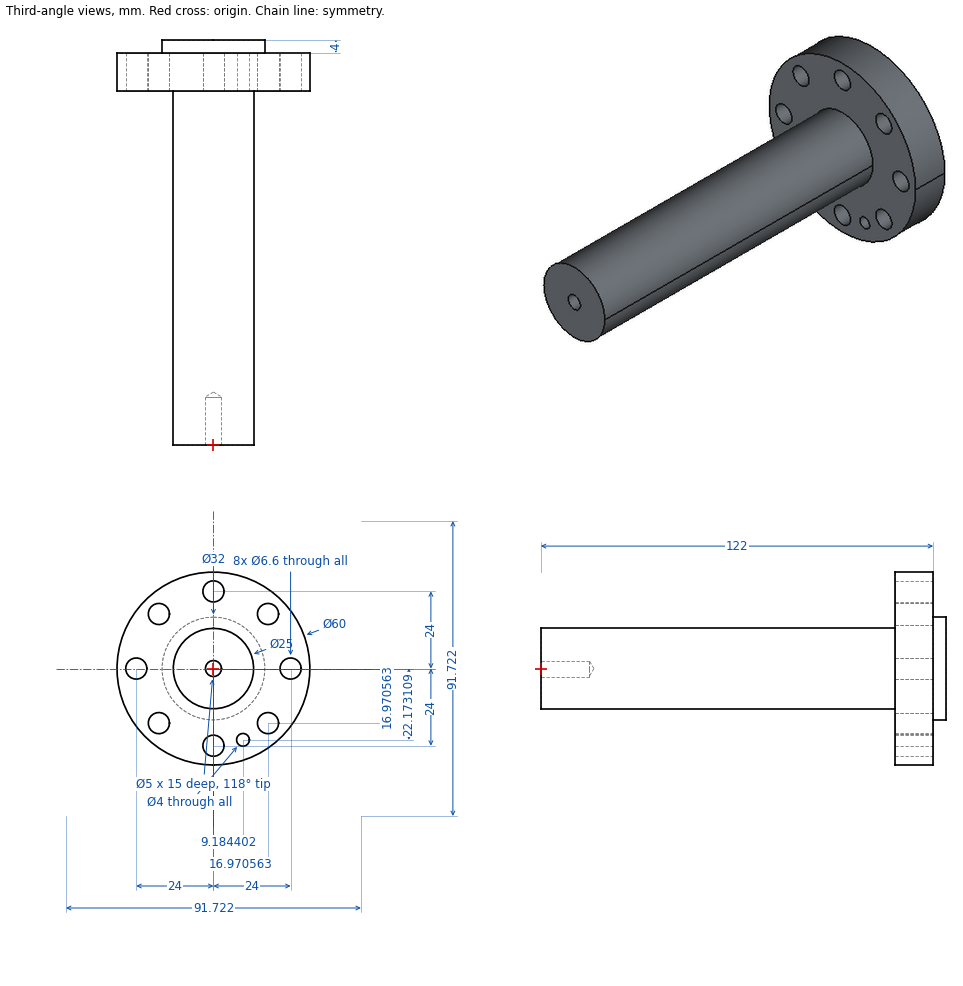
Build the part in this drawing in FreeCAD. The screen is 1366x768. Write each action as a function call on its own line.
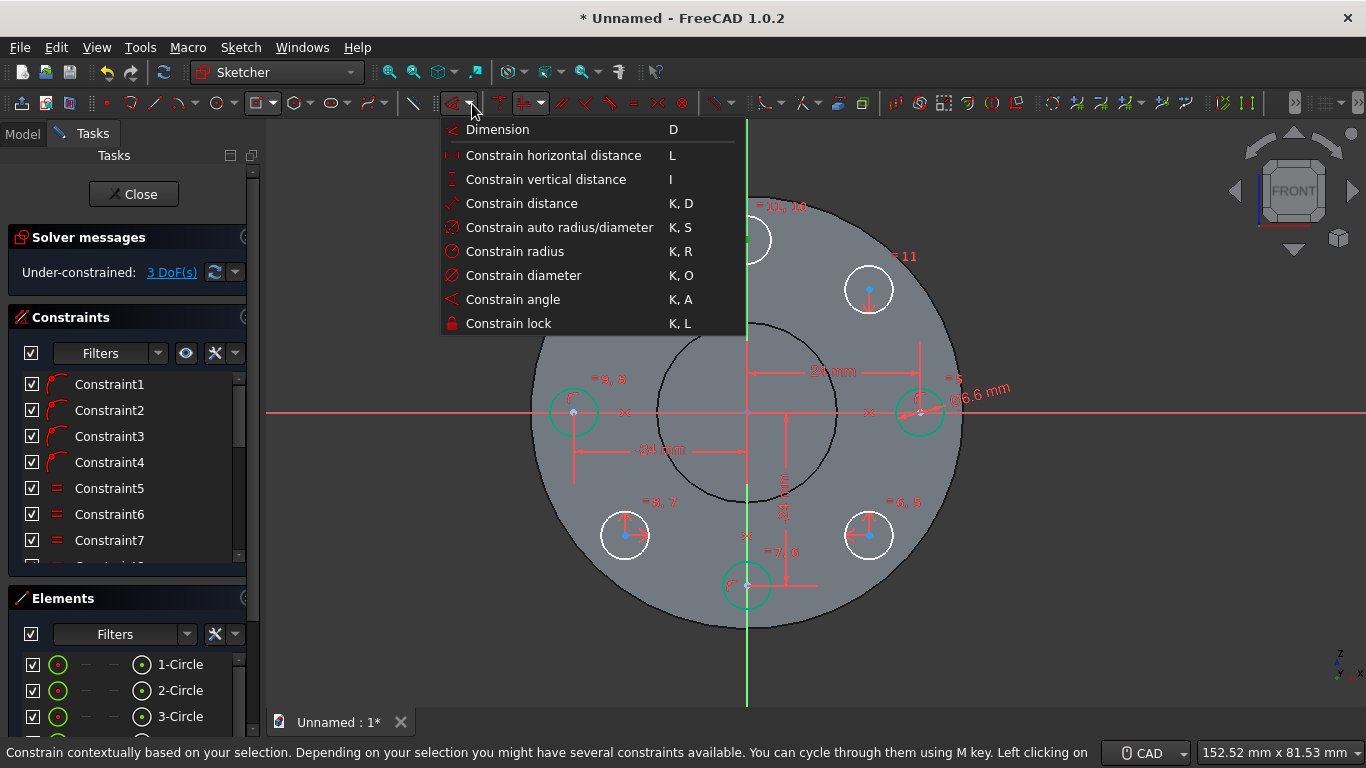
click(593, 179)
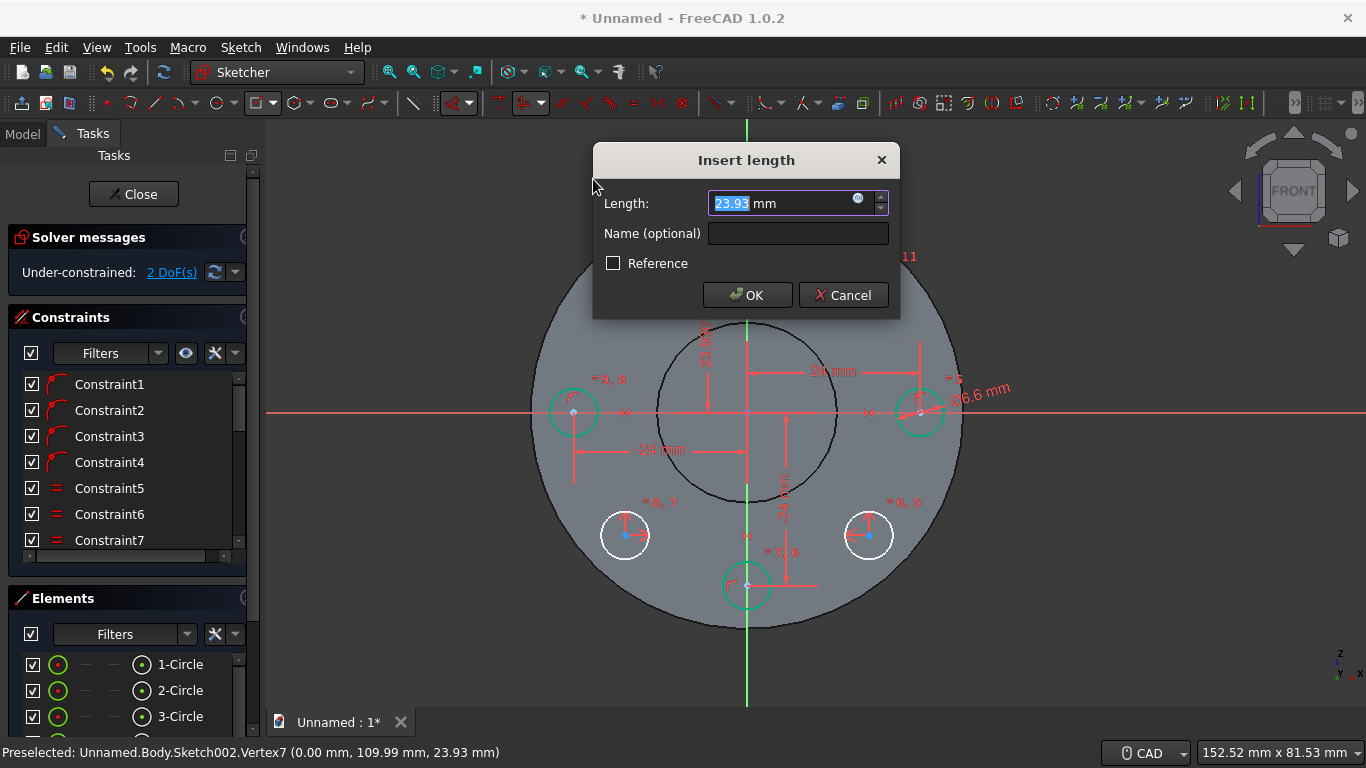
text(24)
key(Return)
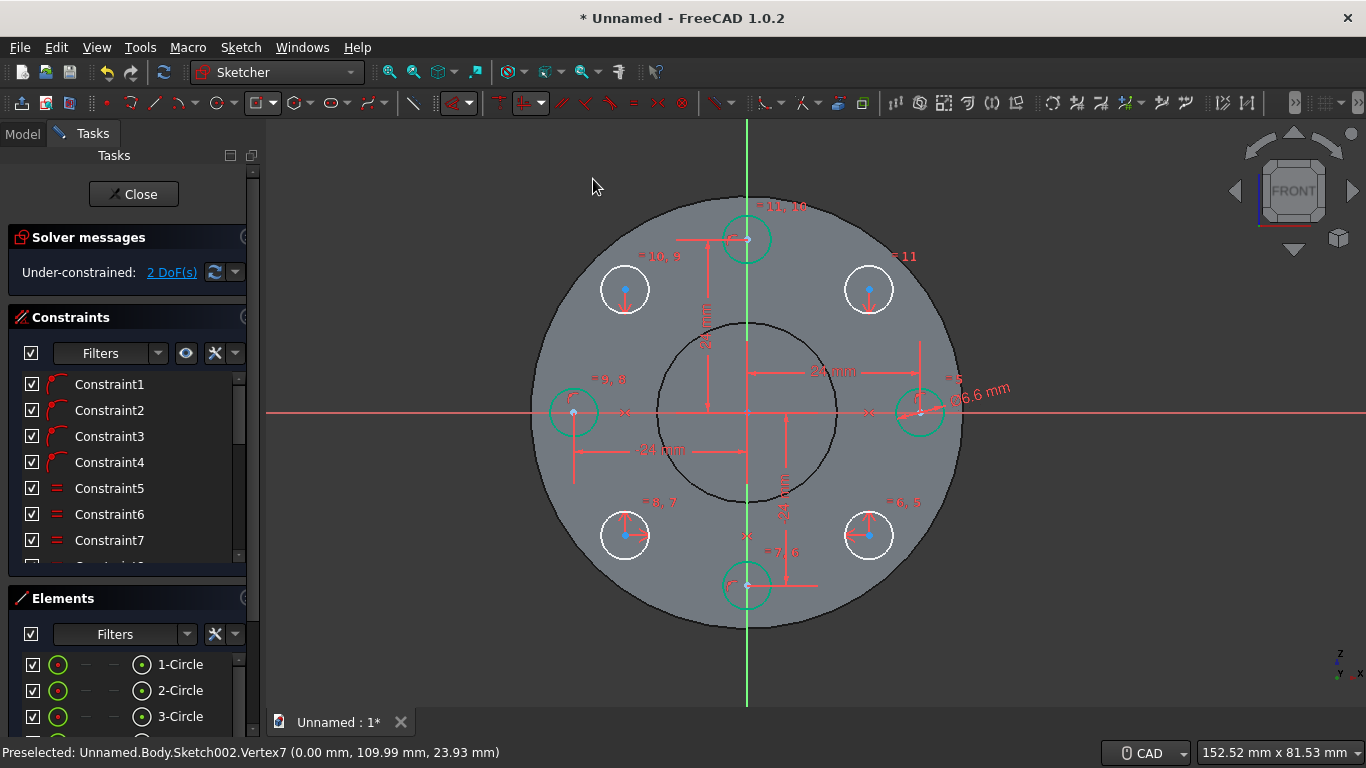
click(869, 535)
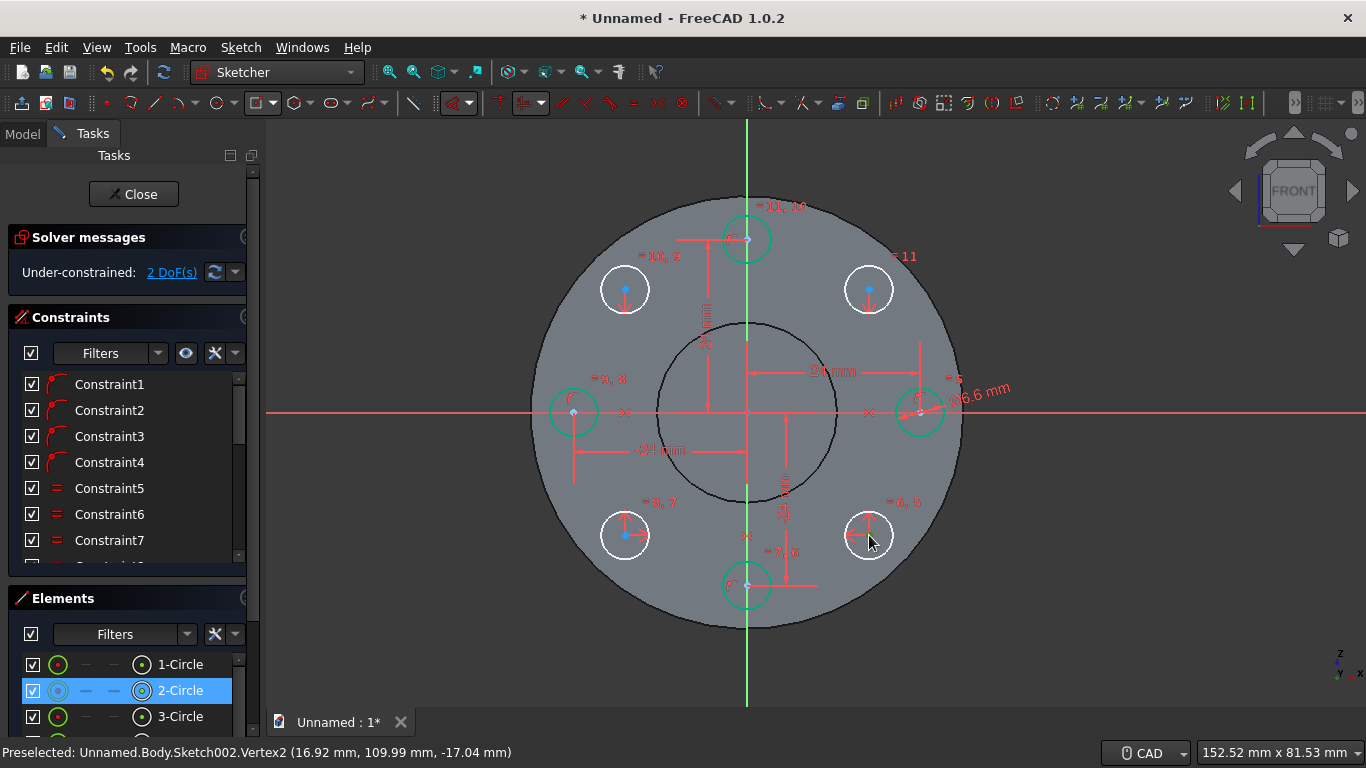
key(l)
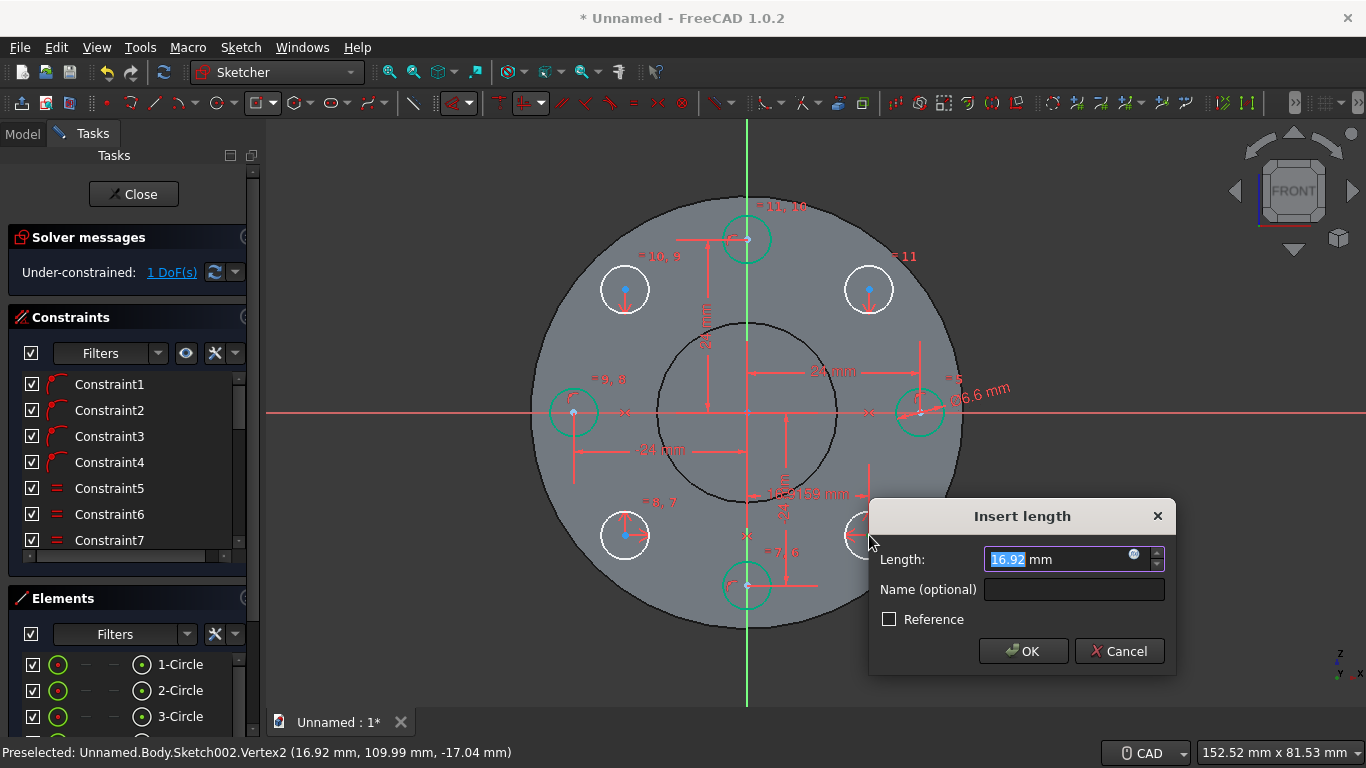
text(16.970563)
key(Return)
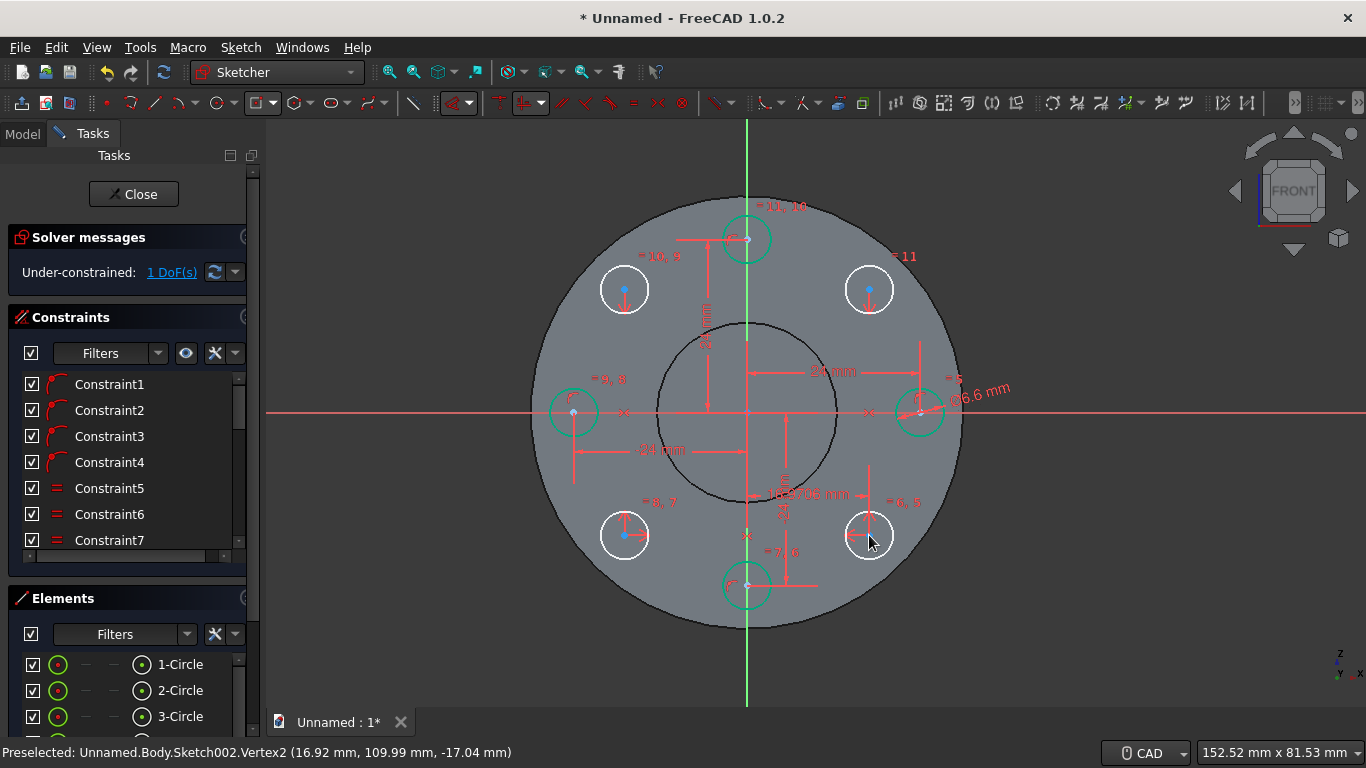
click(869, 535)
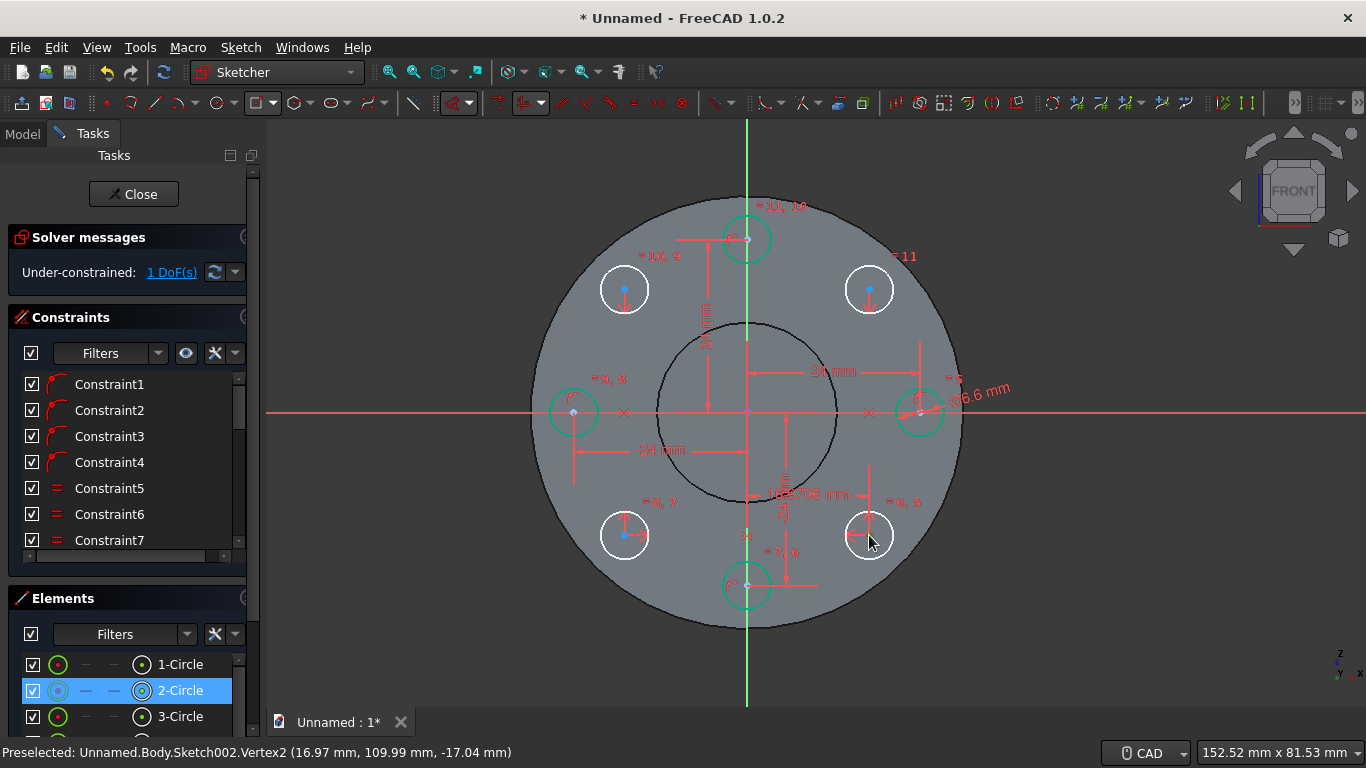
click(472, 104)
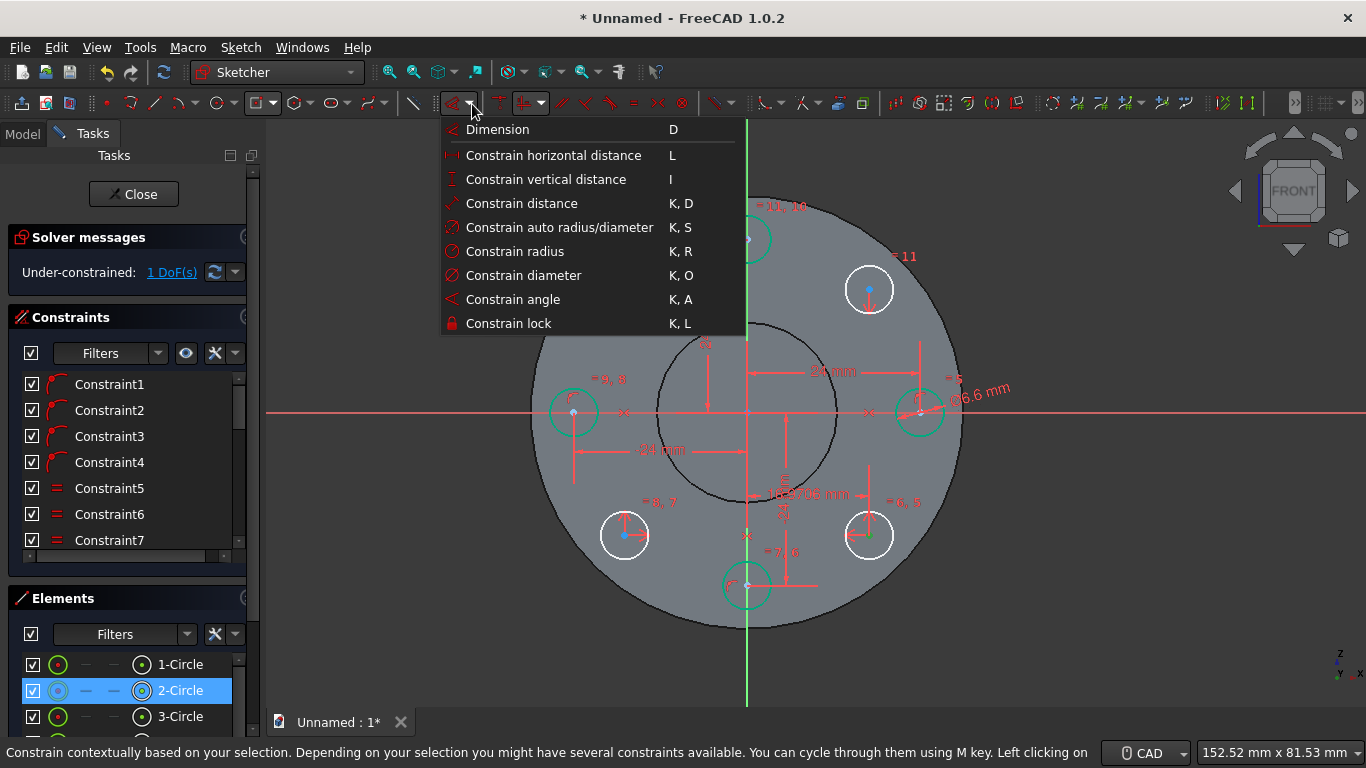
click(593, 179)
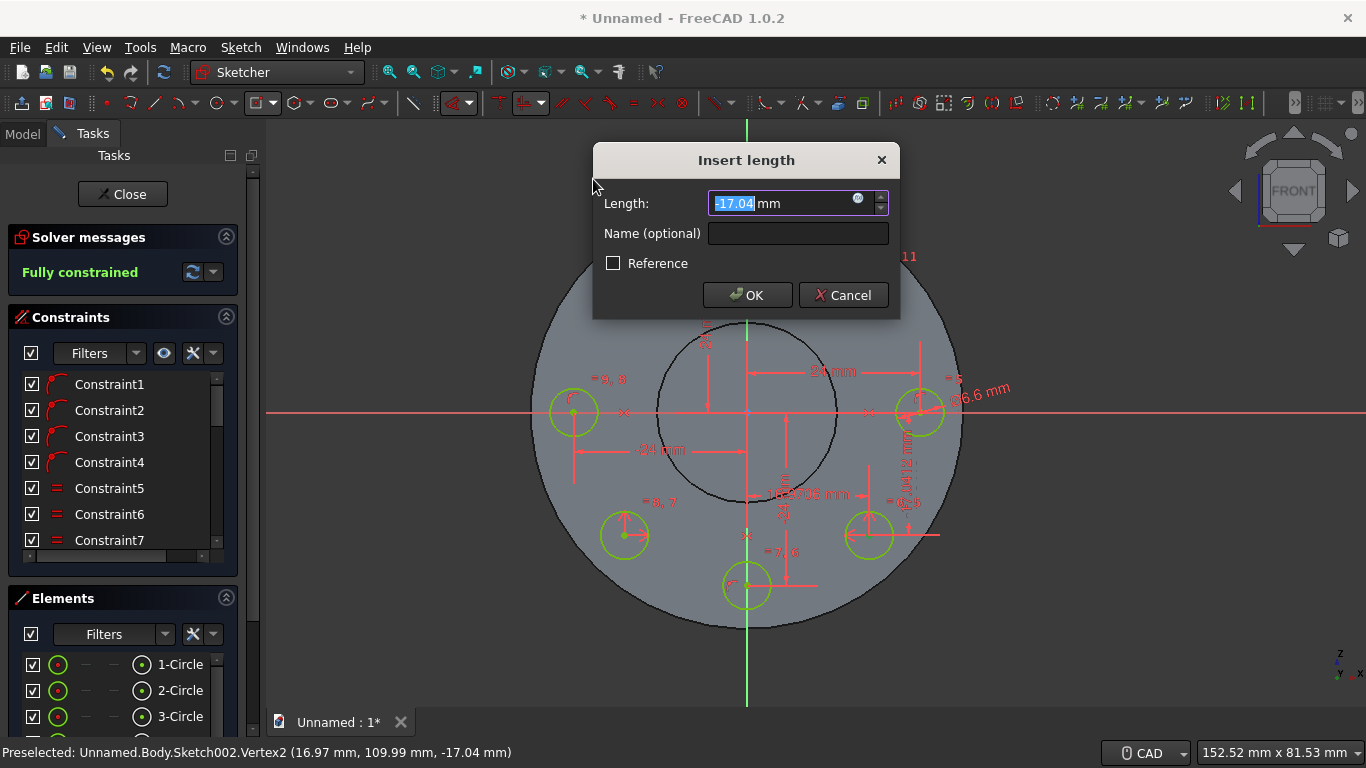
text(-16.970563)
key(Return)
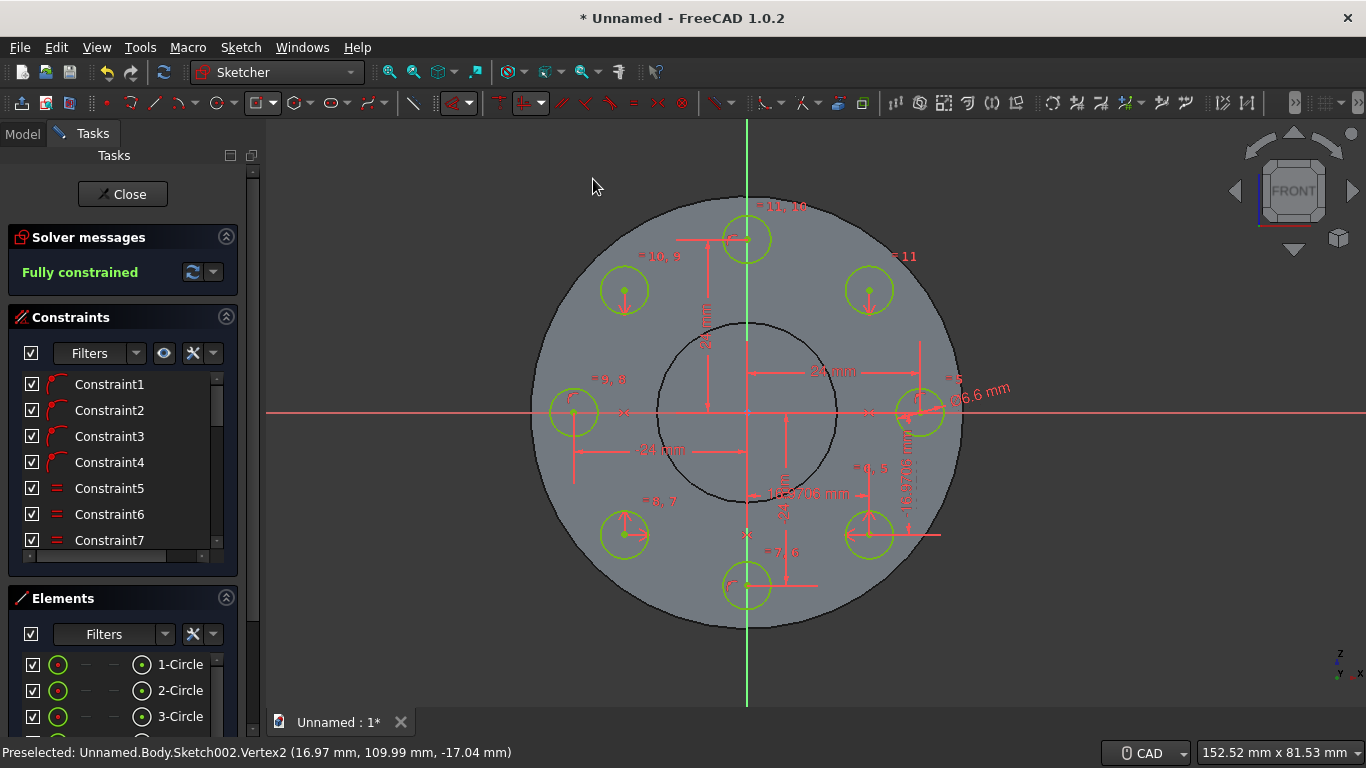
click(123, 194)